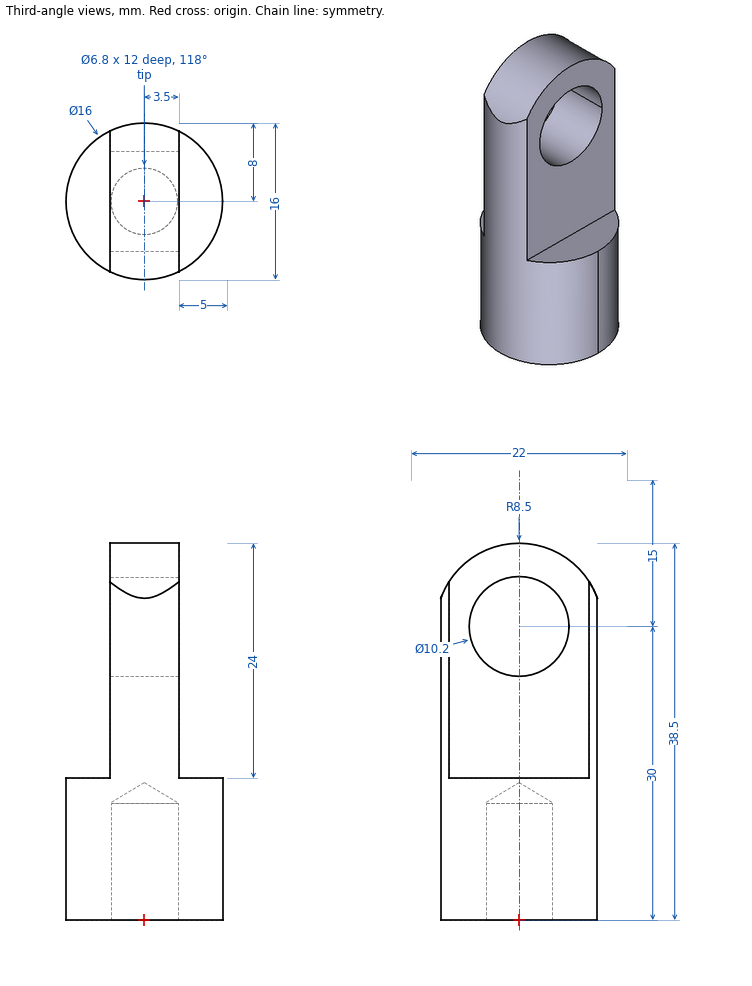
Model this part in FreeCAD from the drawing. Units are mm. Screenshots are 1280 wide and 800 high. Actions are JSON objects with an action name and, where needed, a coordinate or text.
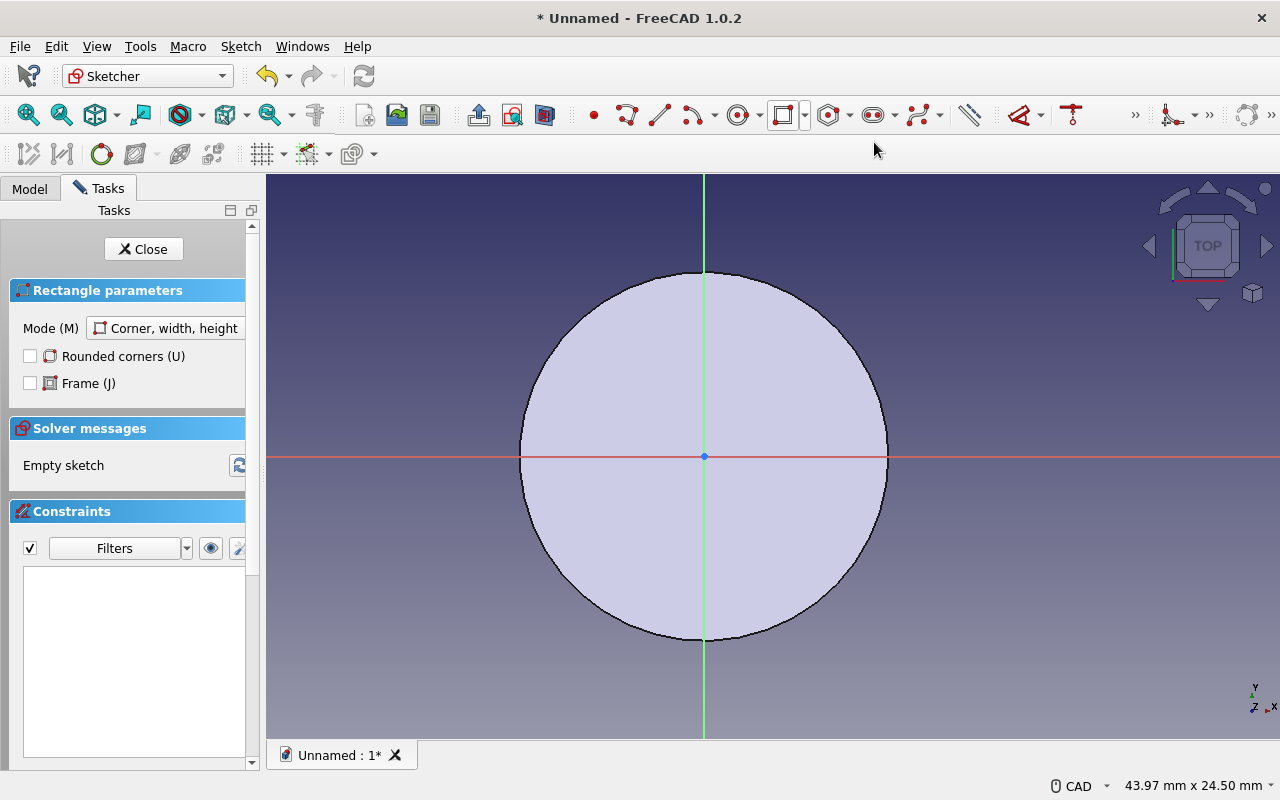
{"action": "left_click", "coordinate": [785, 272]}
{"action": "left_click", "coordinate": [900, 641]}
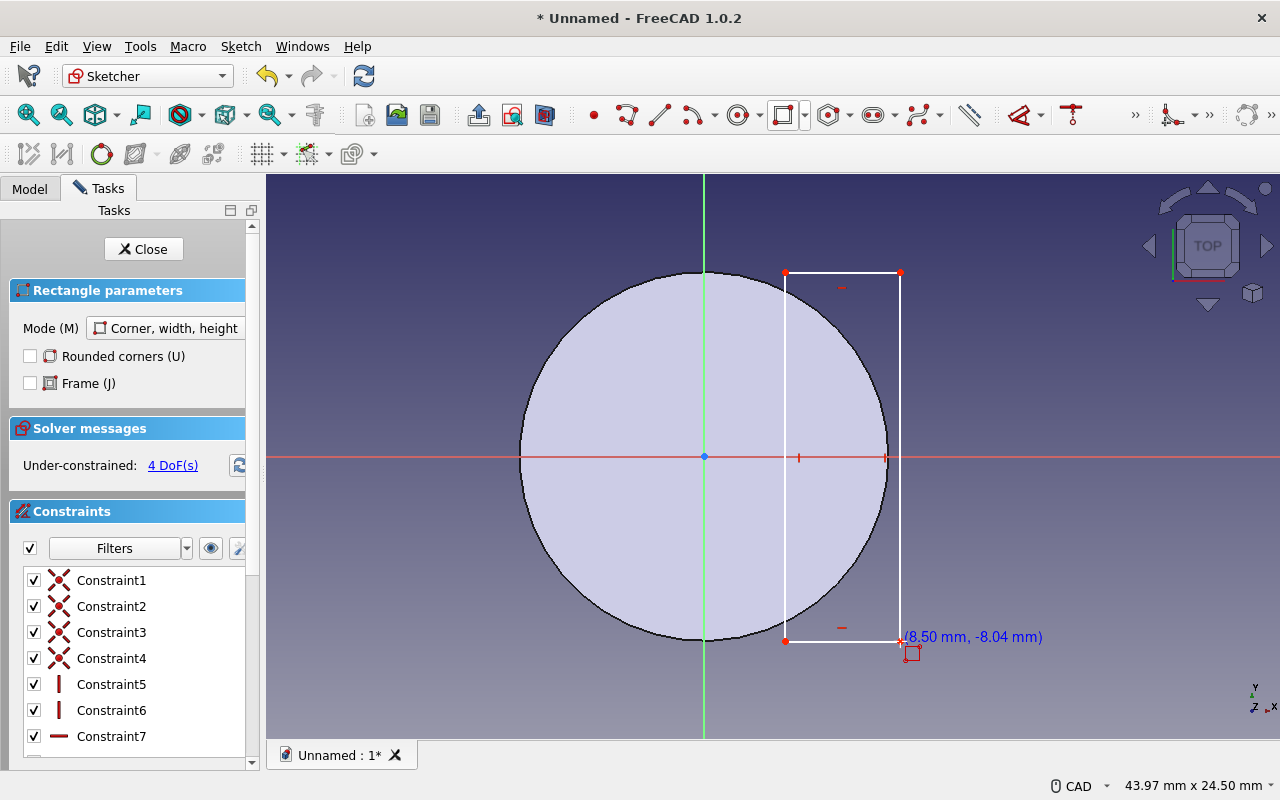
{"action": "left_click", "coordinate": [508, 272]}
{"action": "left_click", "coordinate": [623, 641]}
{"action": "key", "text": "Escape"}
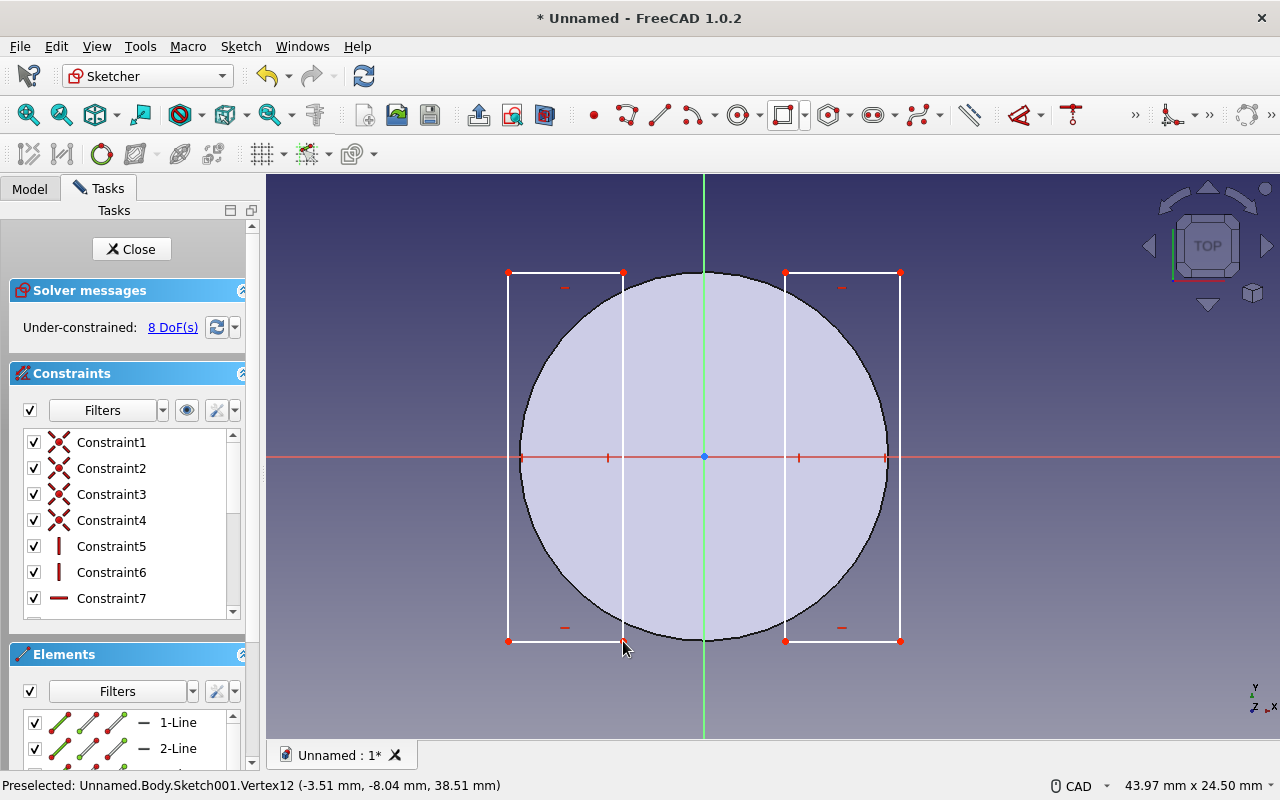
{"action": "left_click", "coordinate": [900, 273]}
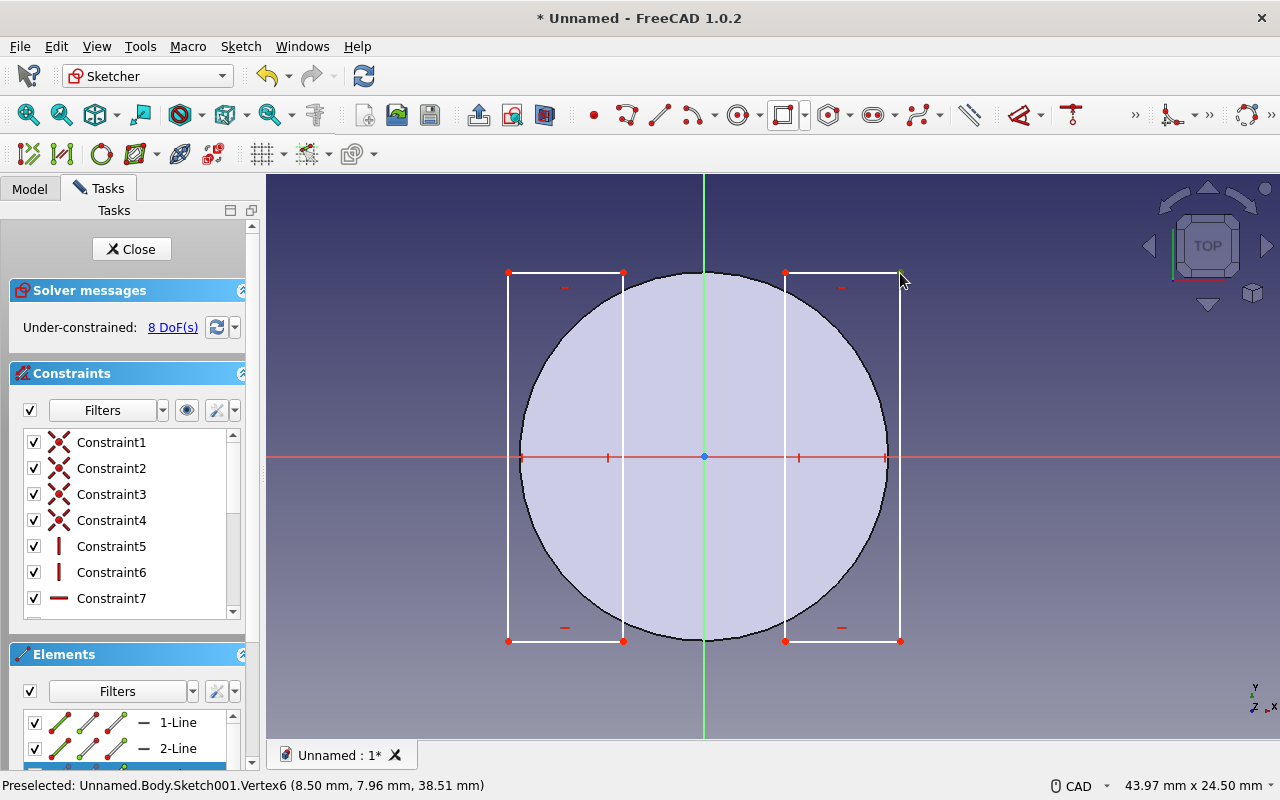
{"action": "left_click", "coordinate": [508, 273]}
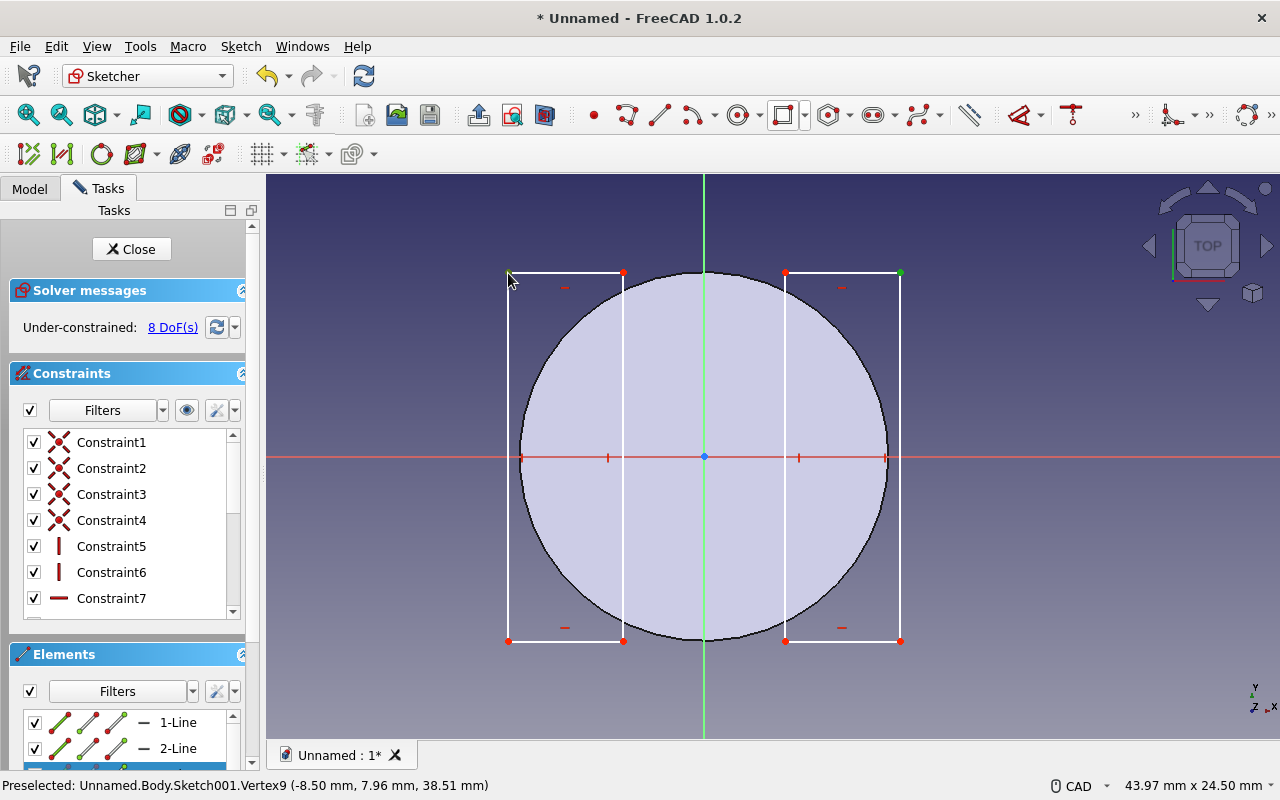
{"action": "left_click", "coordinate": [704, 675]}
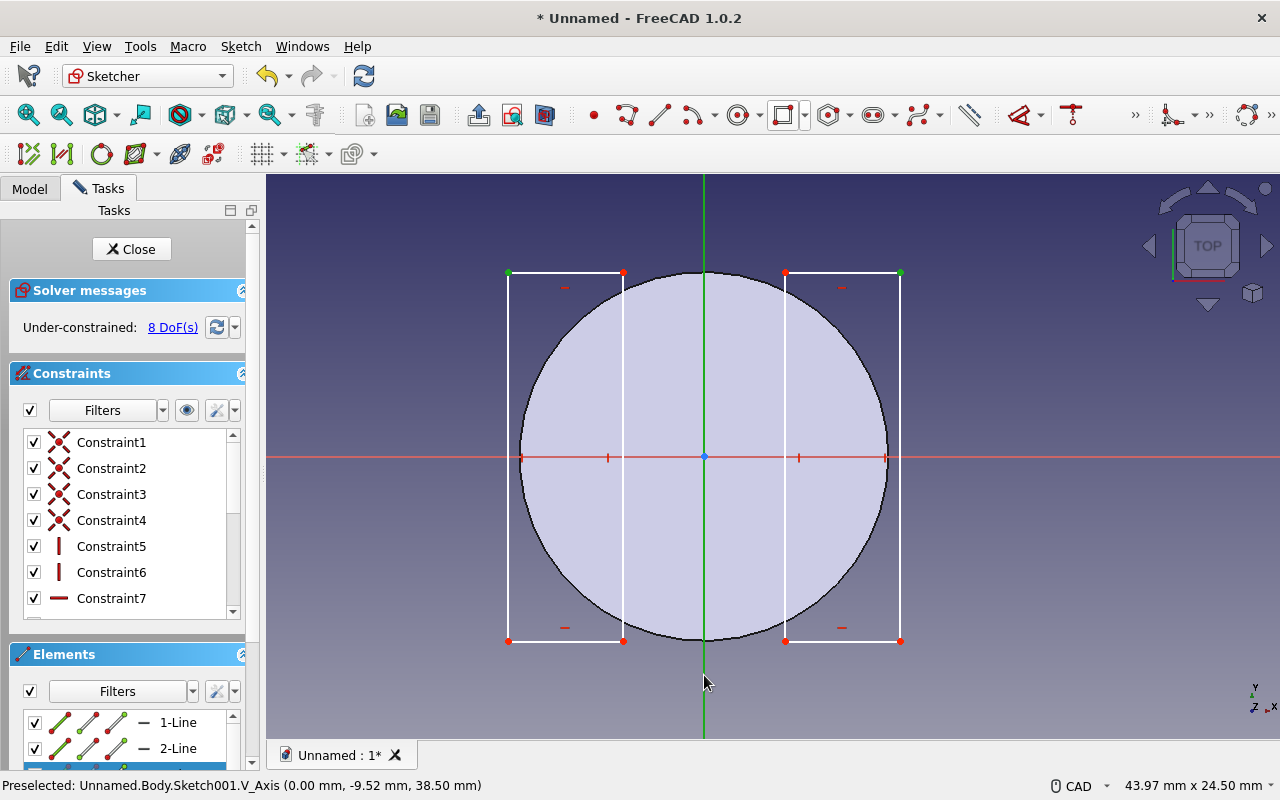
{"action": "key", "text": "s"}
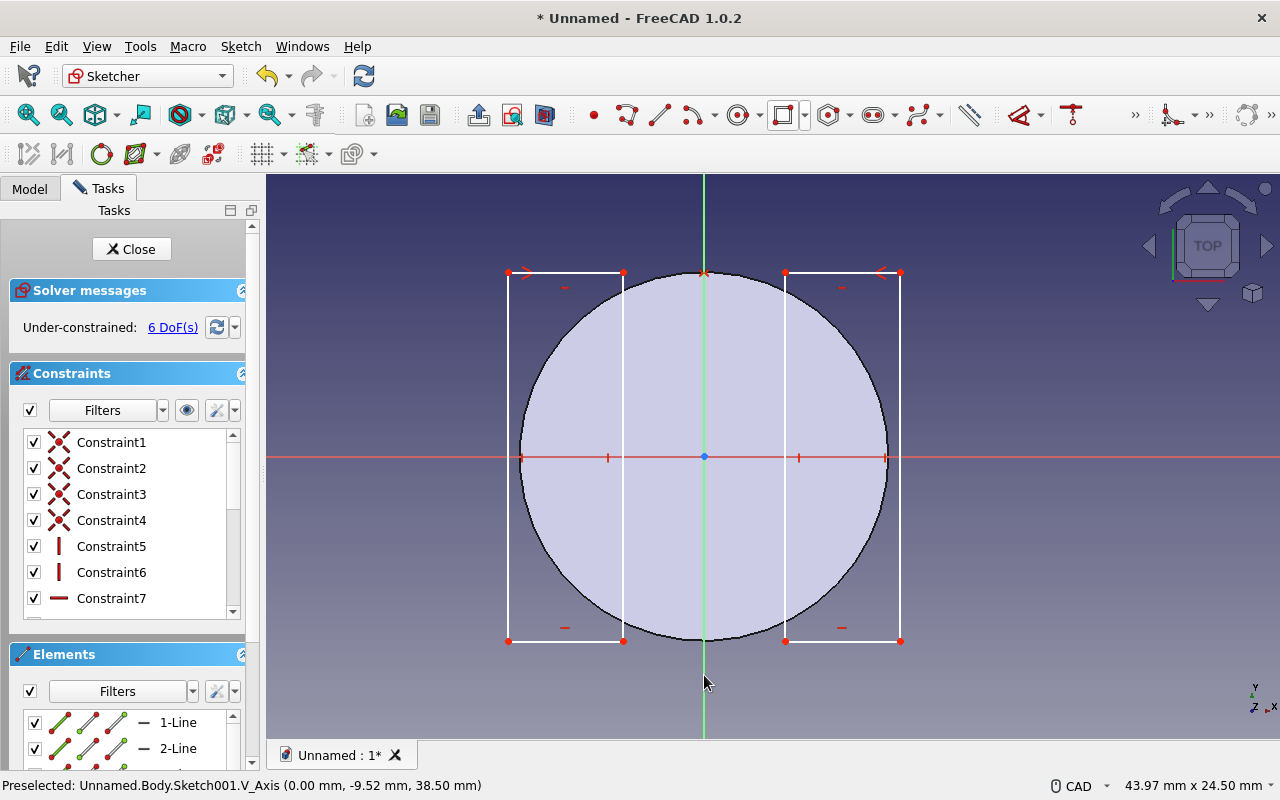
{"action": "left_click", "coordinate": [785, 642]}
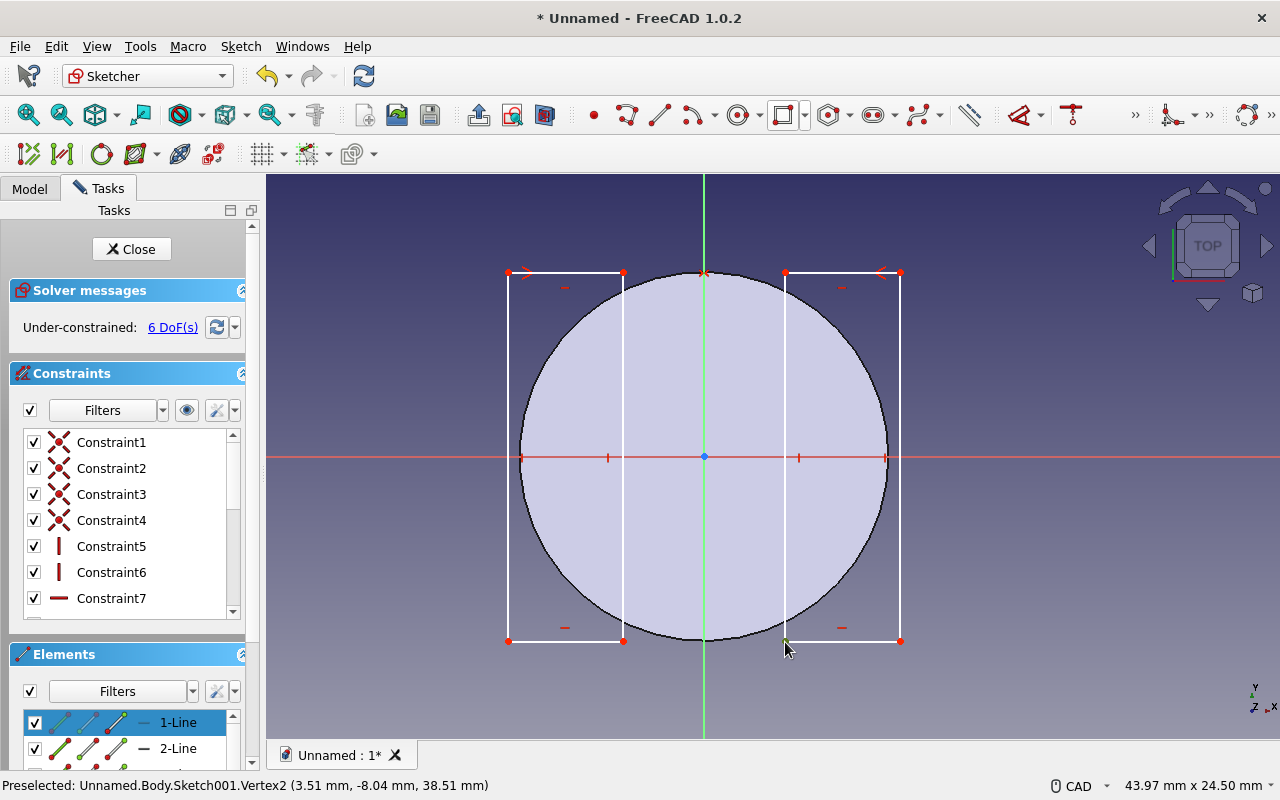
{"action": "left_click", "coordinate": [623, 642]}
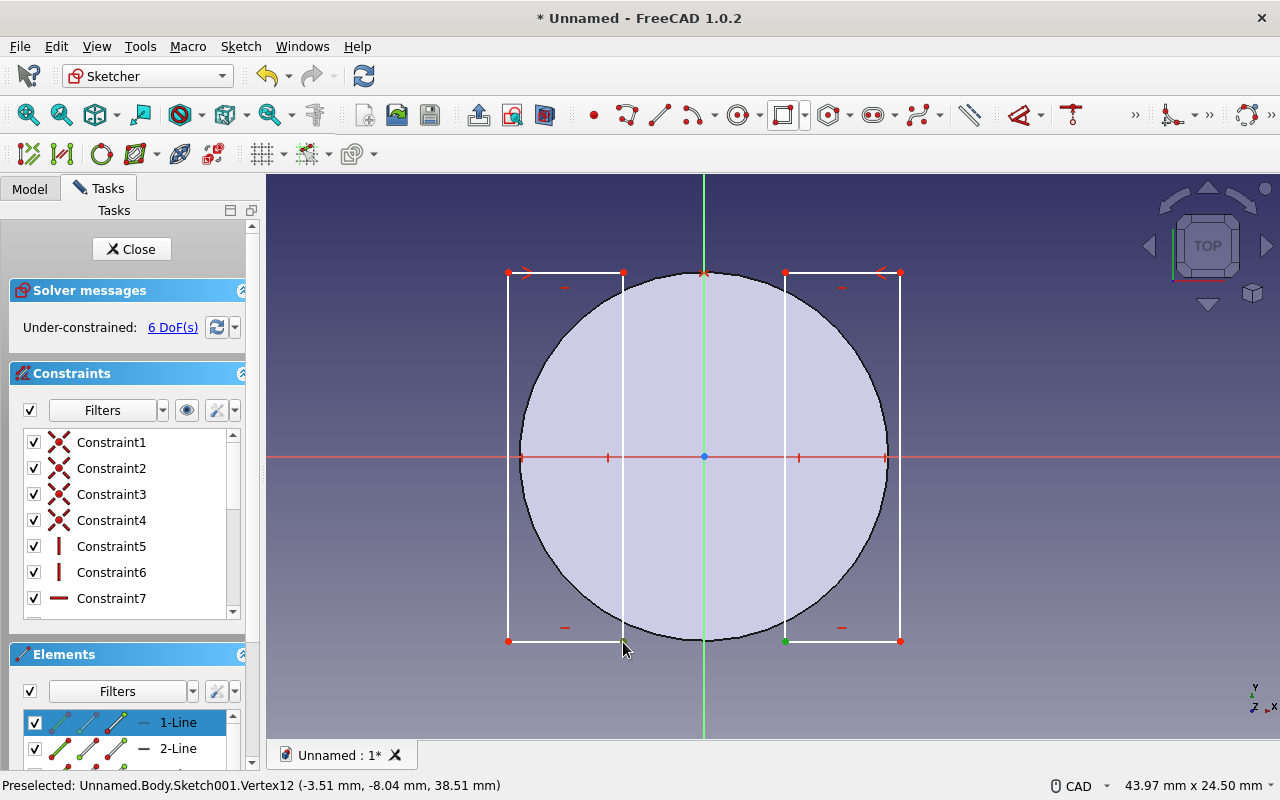
{"action": "left_click", "coordinate": [704, 675]}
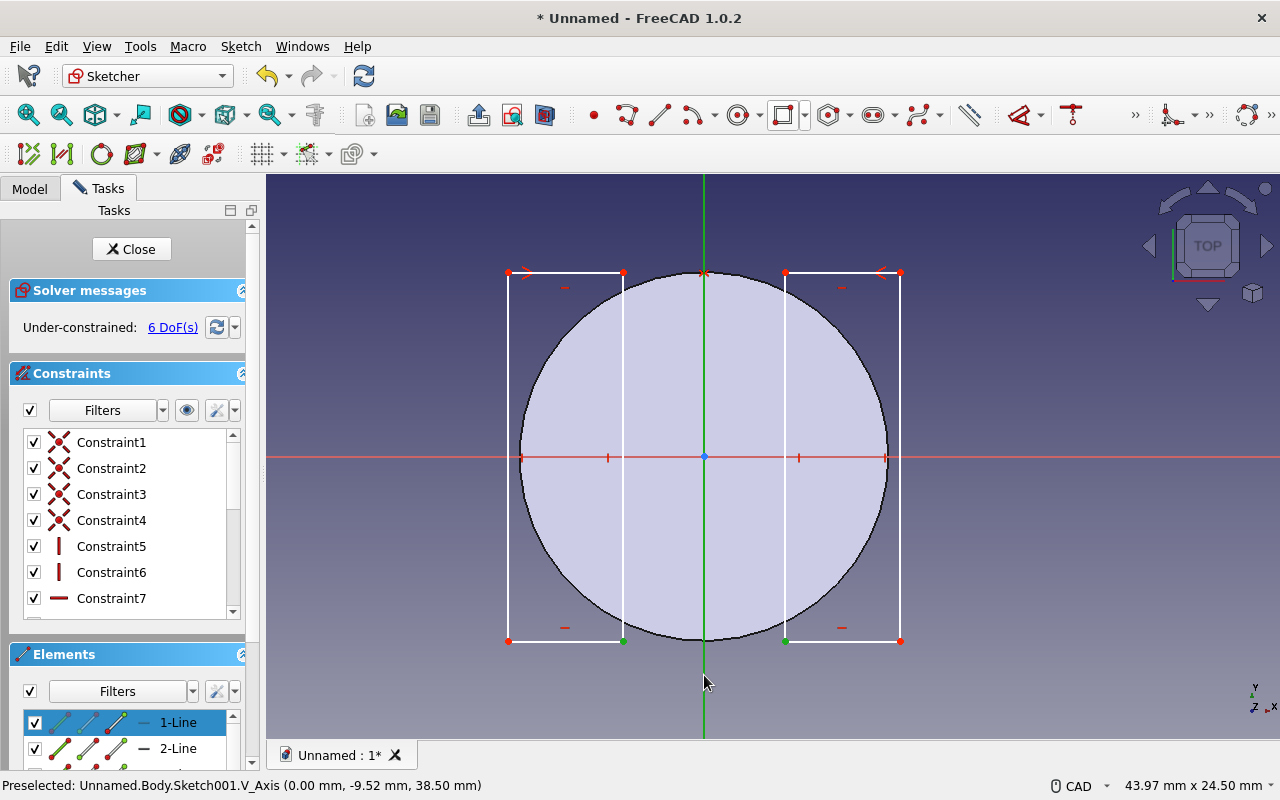
{"action": "key", "text": "s"}